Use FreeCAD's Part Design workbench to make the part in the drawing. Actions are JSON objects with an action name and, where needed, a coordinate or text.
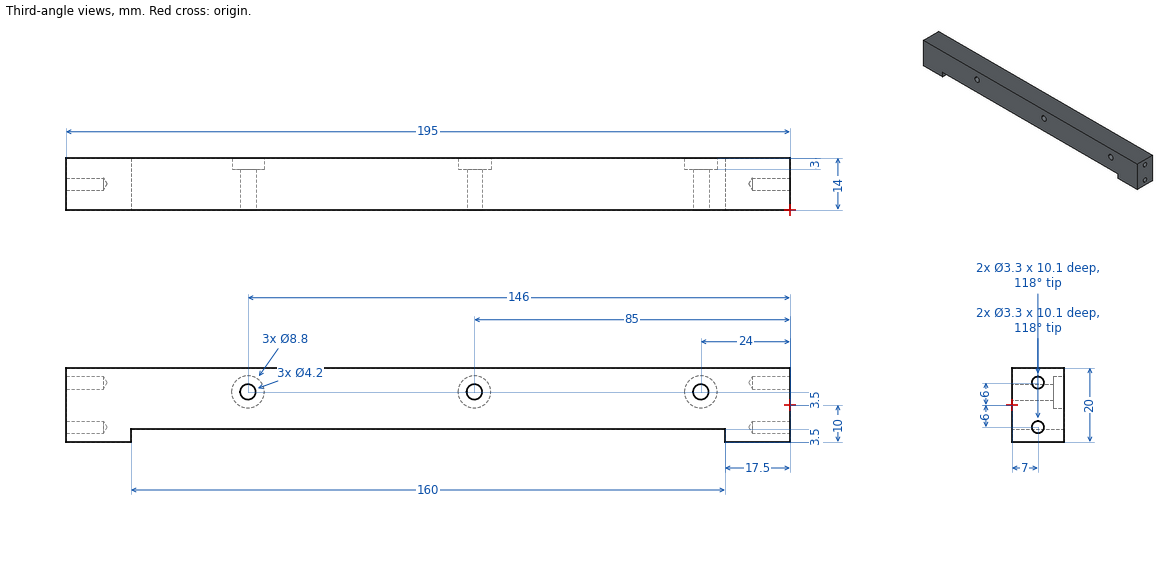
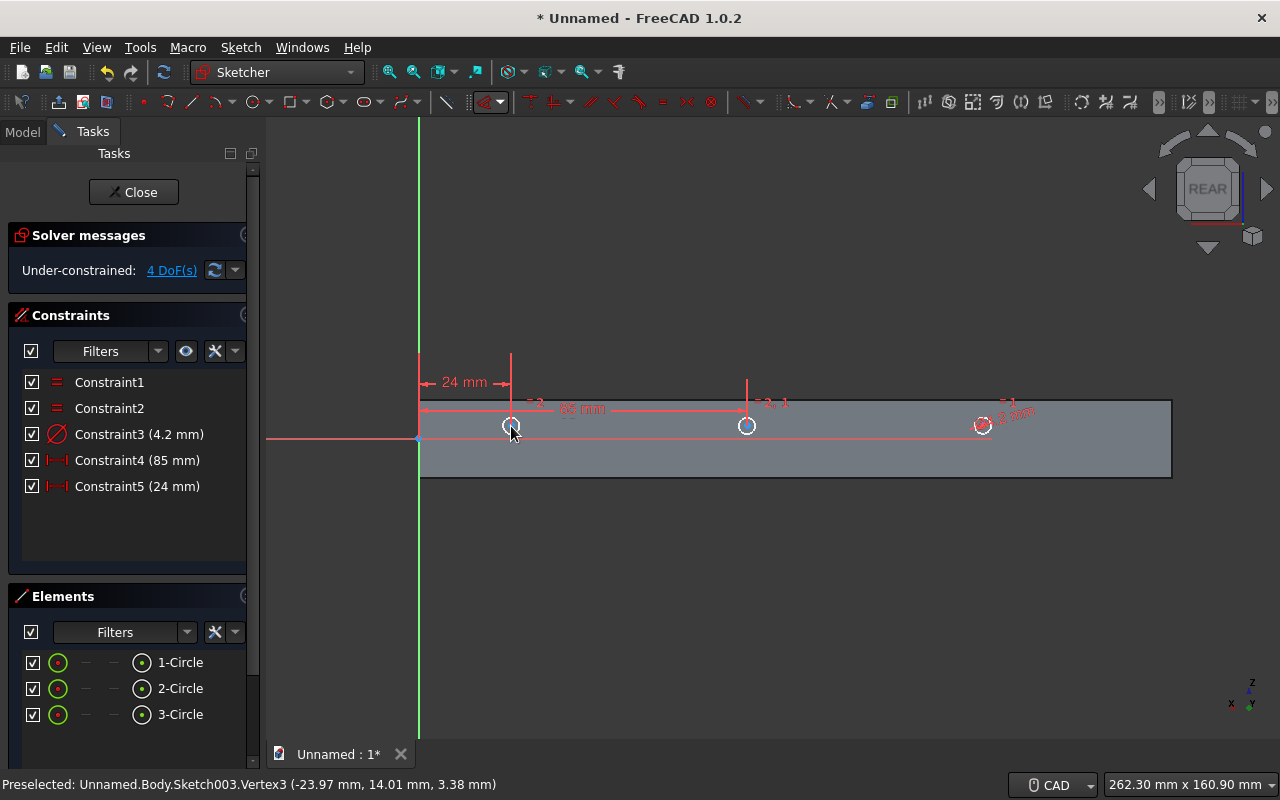
{"action": "left_click", "coordinate": [983, 426]}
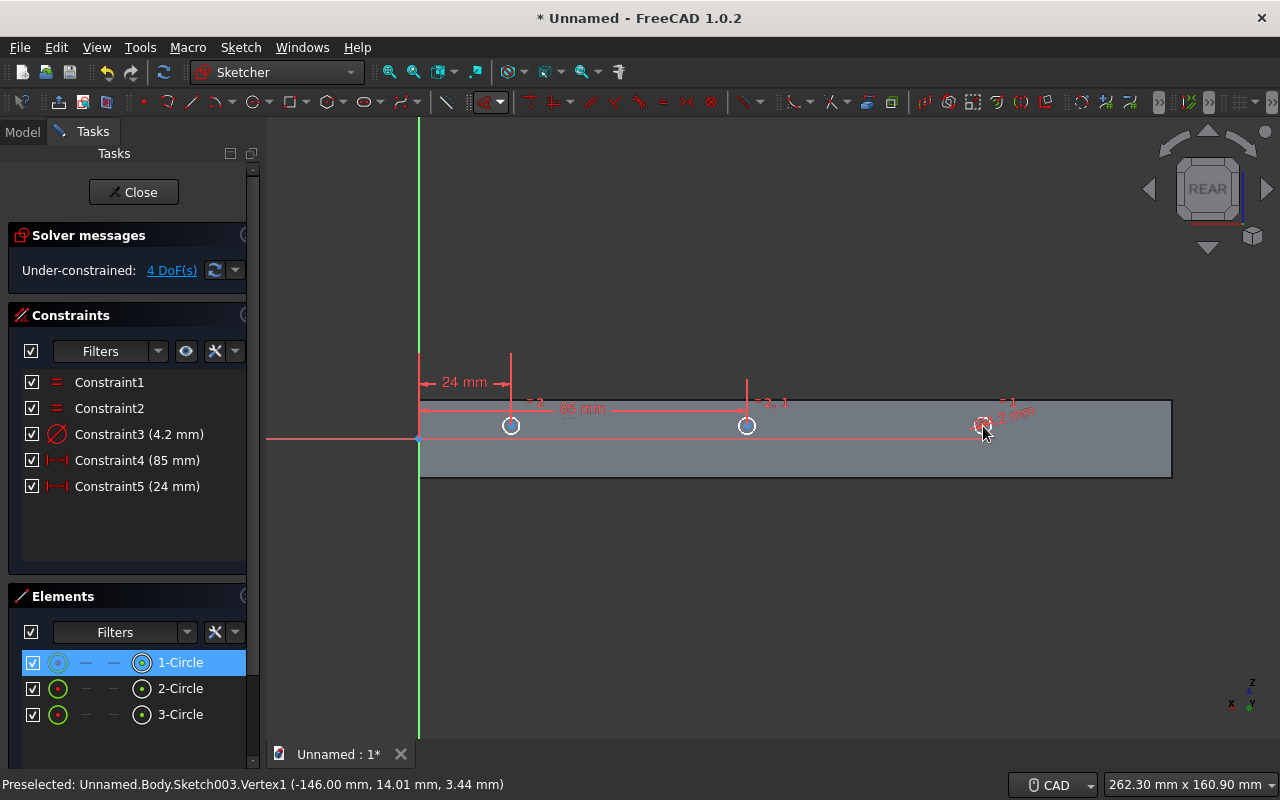
{"action": "key", "text": "l"}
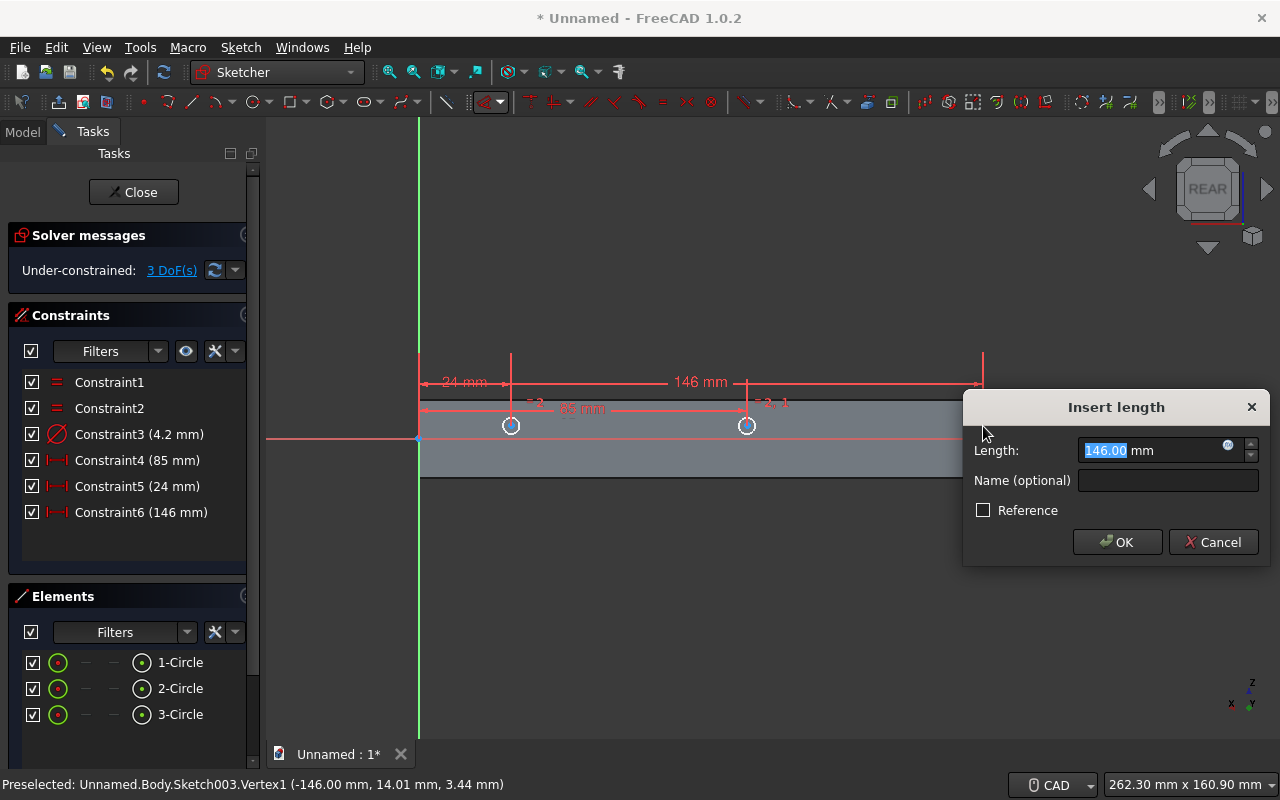
{"action": "type", "text": "146"}
{"action": "key", "text": "Return"}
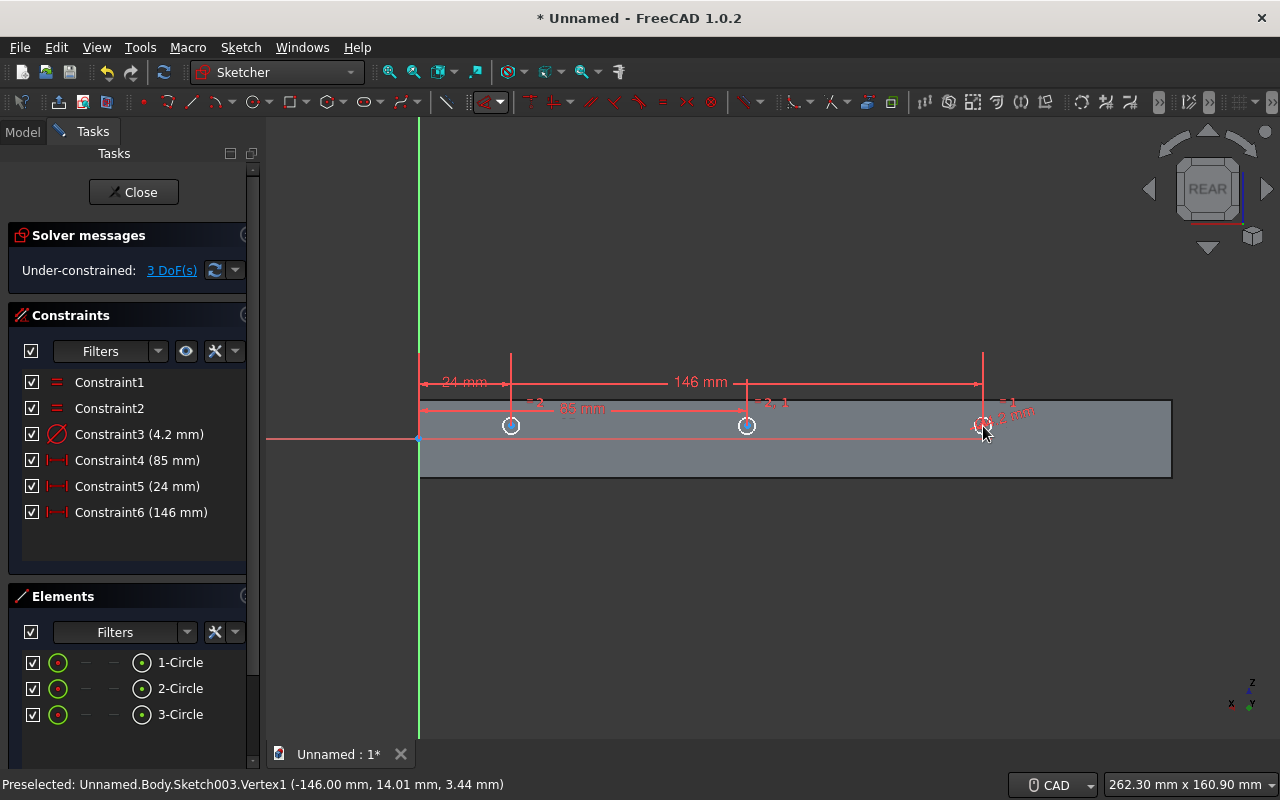
{"action": "scroll", "coordinate": [983, 426], "scroll_direction": "up", "scroll_amount": 6}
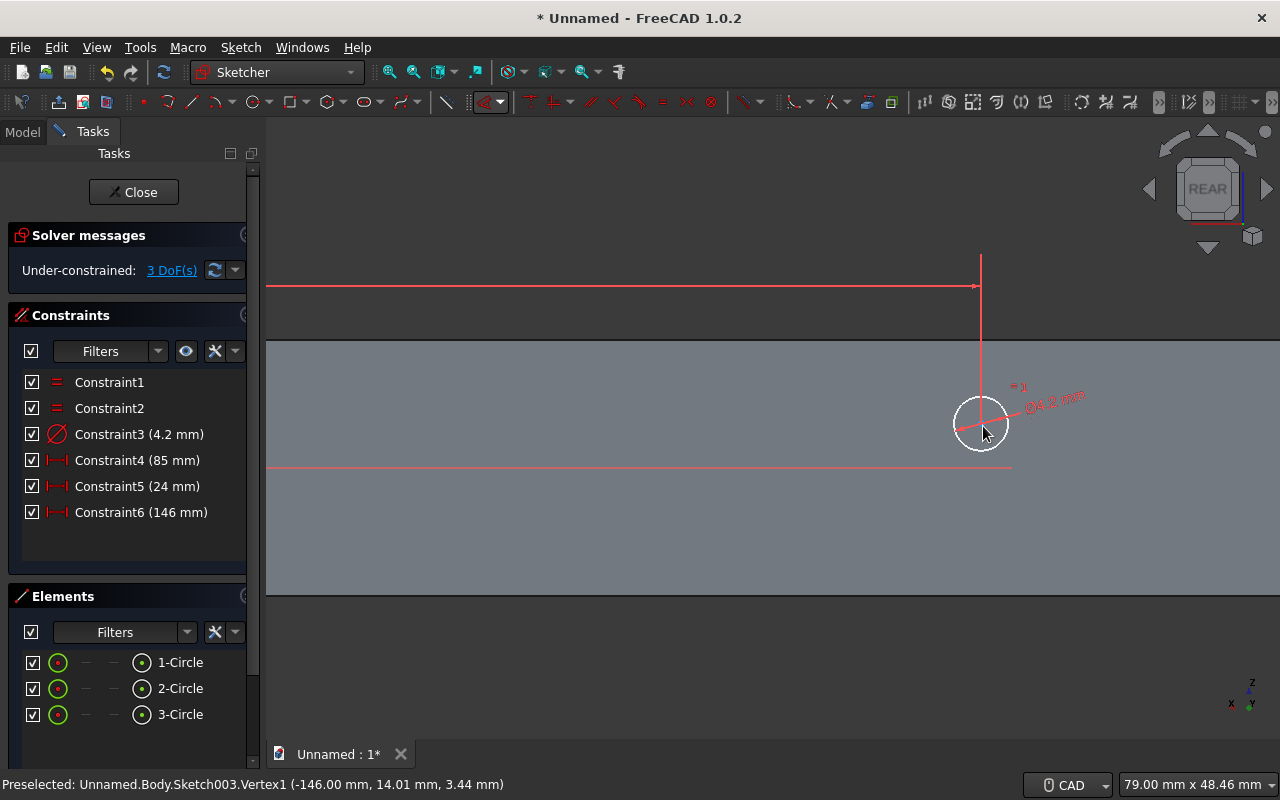
{"action": "left_click", "coordinate": [981, 424]}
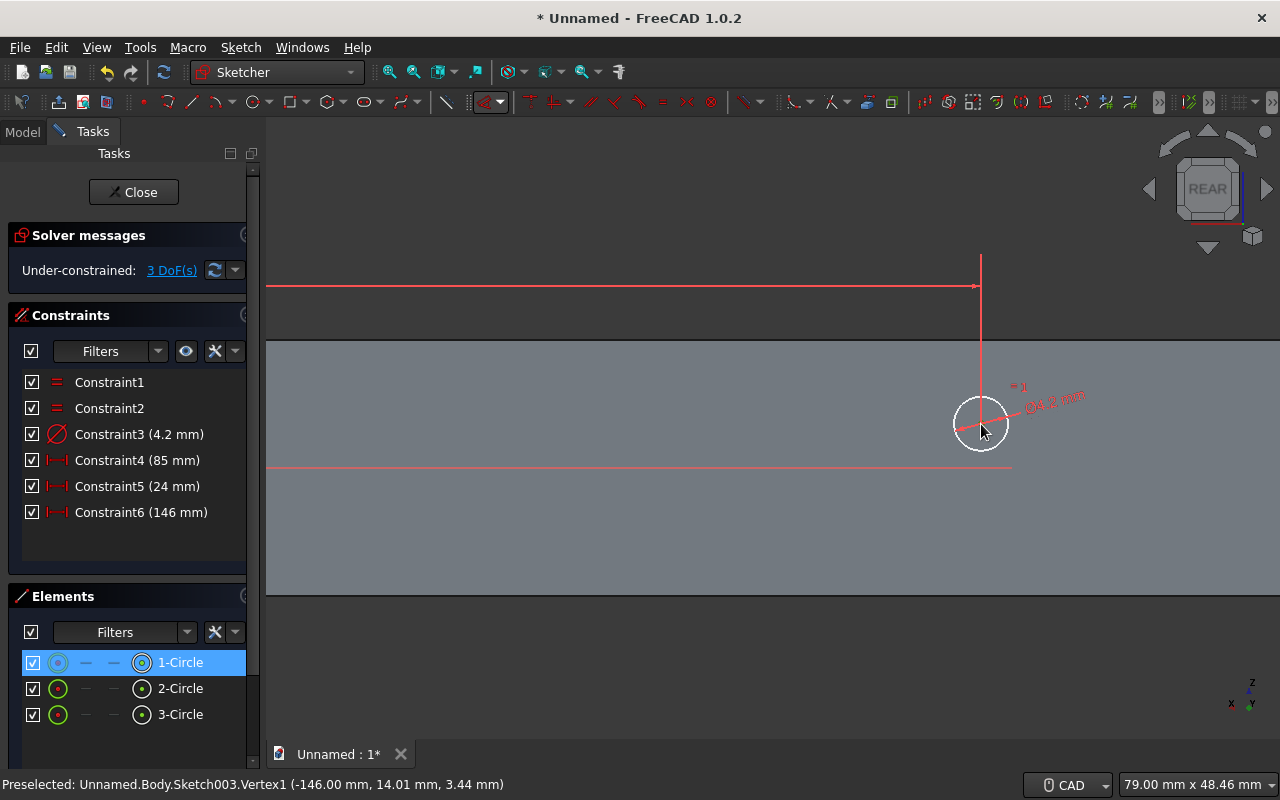
{"action": "key", "text": "i"}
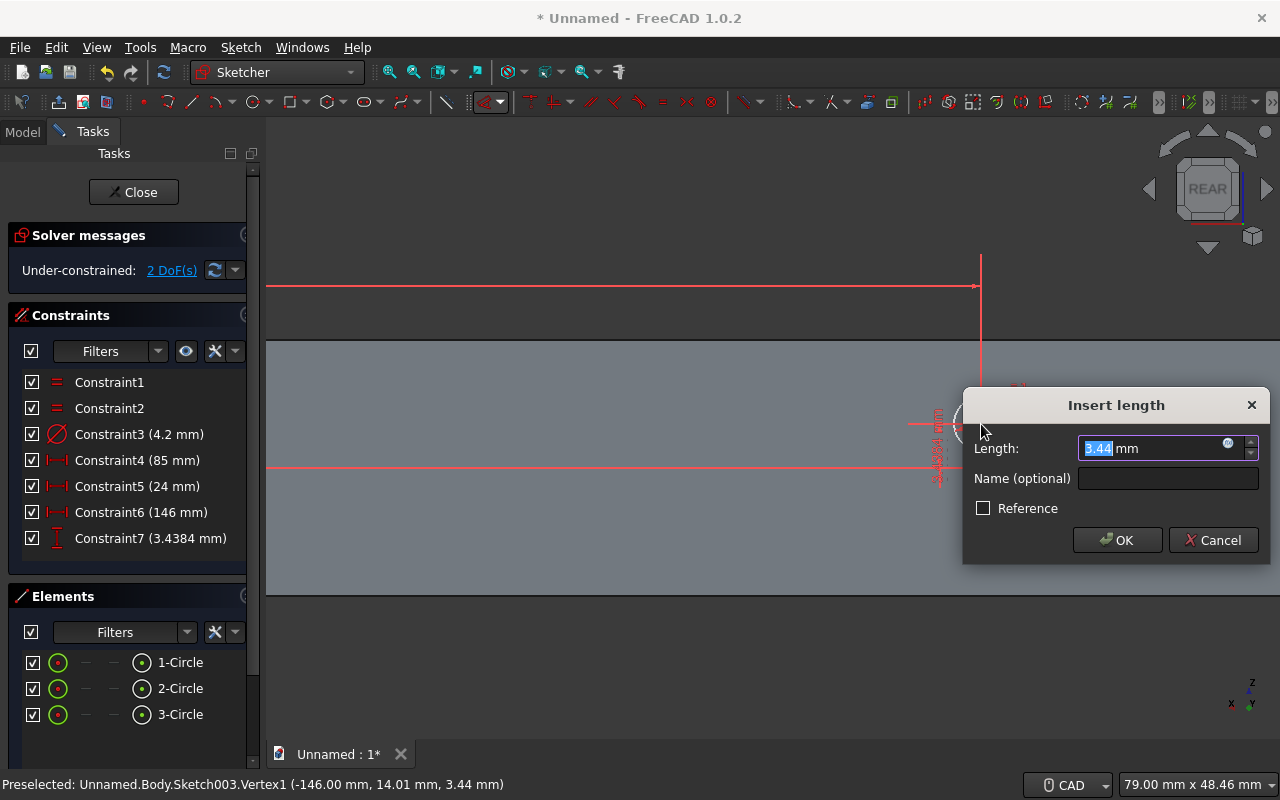
{"action": "type", "text": "3.5"}
{"action": "key", "text": "Return"}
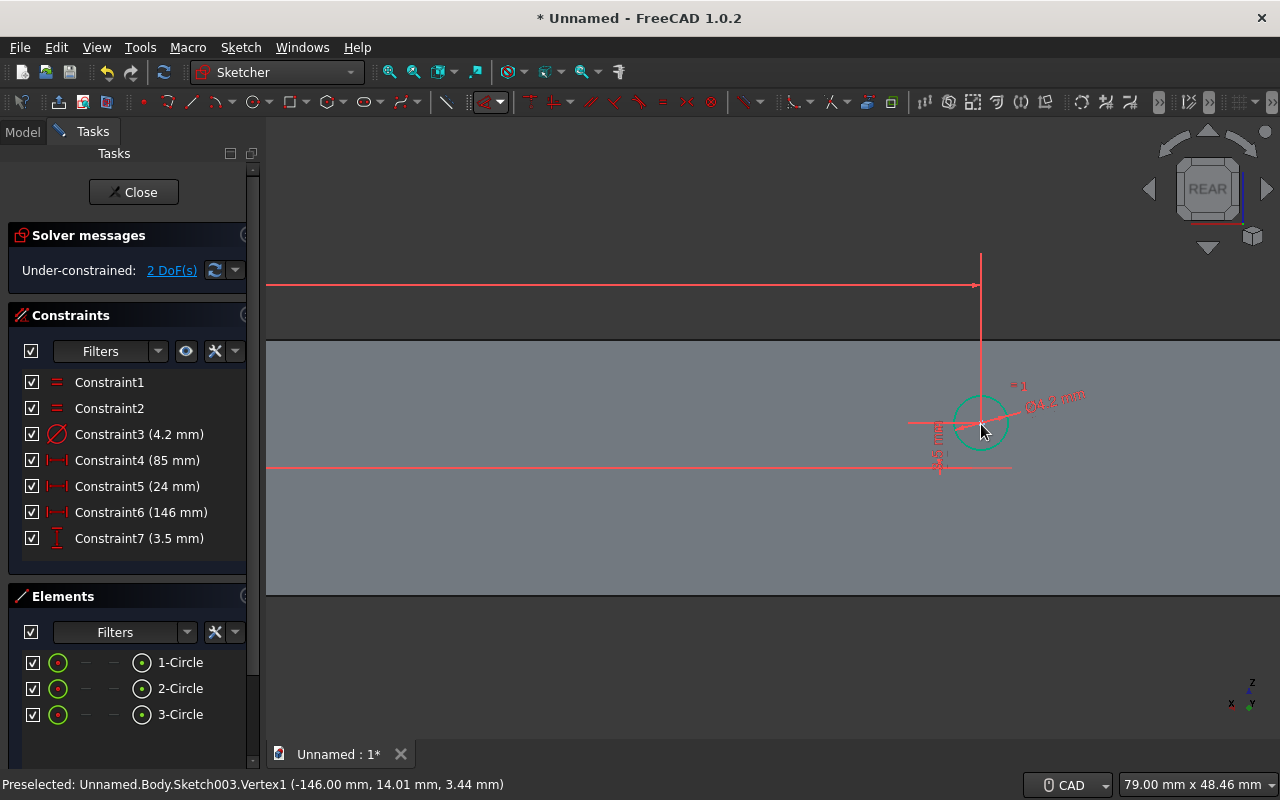
{"action": "scroll", "coordinate": [983, 426], "scroll_direction": "down", "scroll_amount": 6}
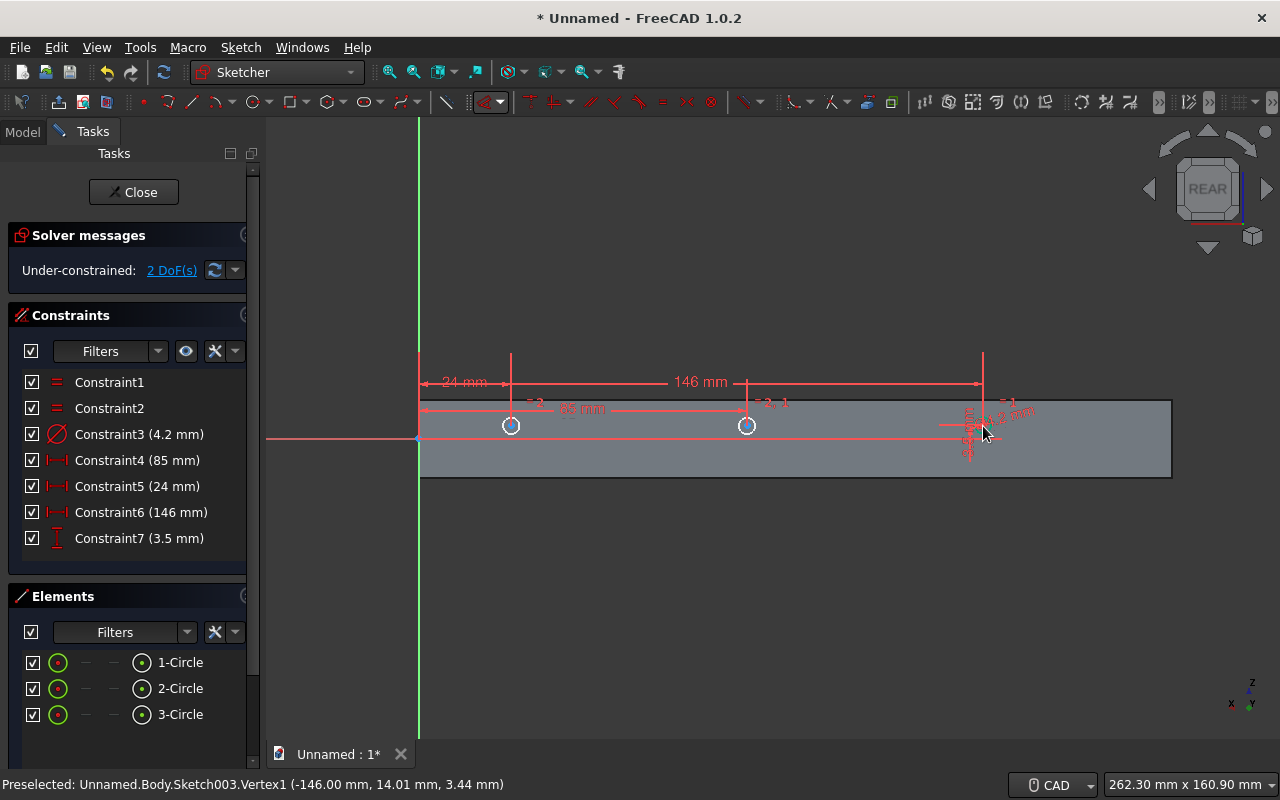
{"action": "scroll", "coordinate": [747, 426], "scroll_direction": "up", "scroll_amount": 6}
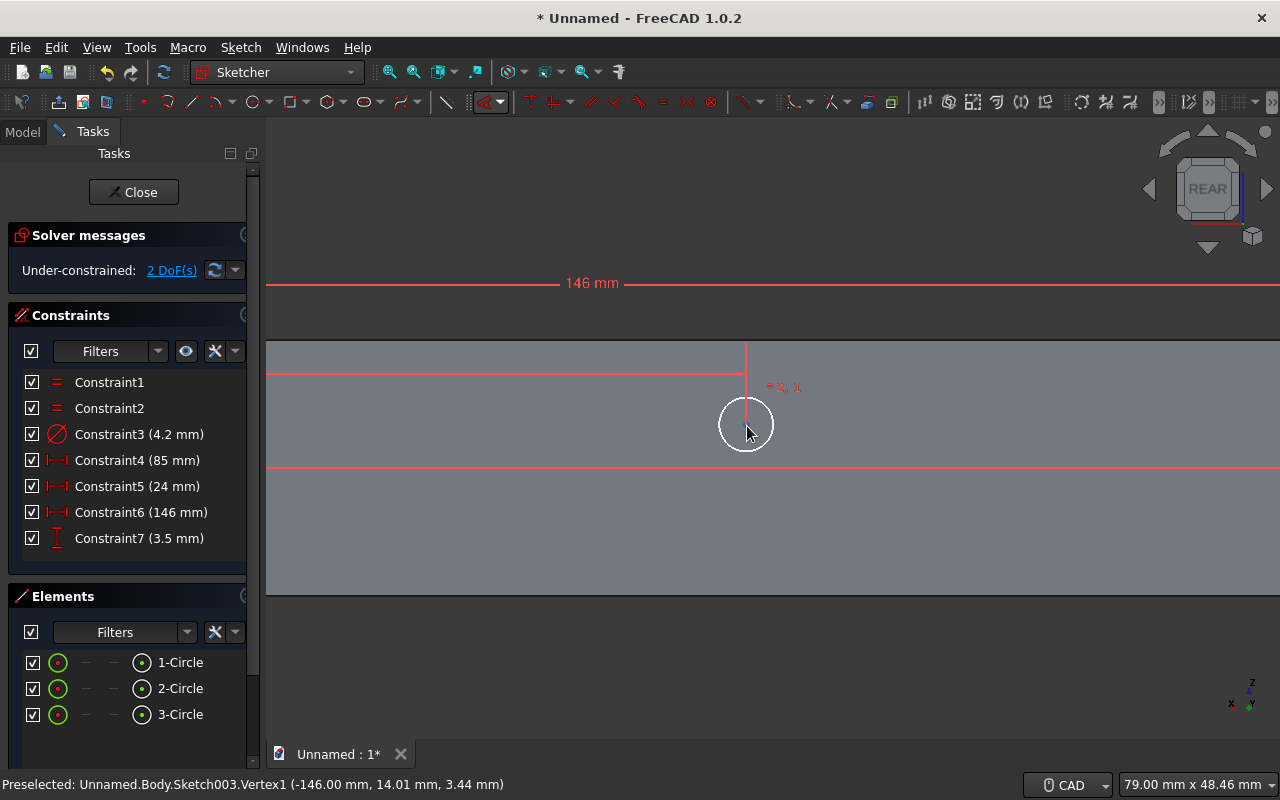
{"action": "left_click", "coordinate": [746, 424]}